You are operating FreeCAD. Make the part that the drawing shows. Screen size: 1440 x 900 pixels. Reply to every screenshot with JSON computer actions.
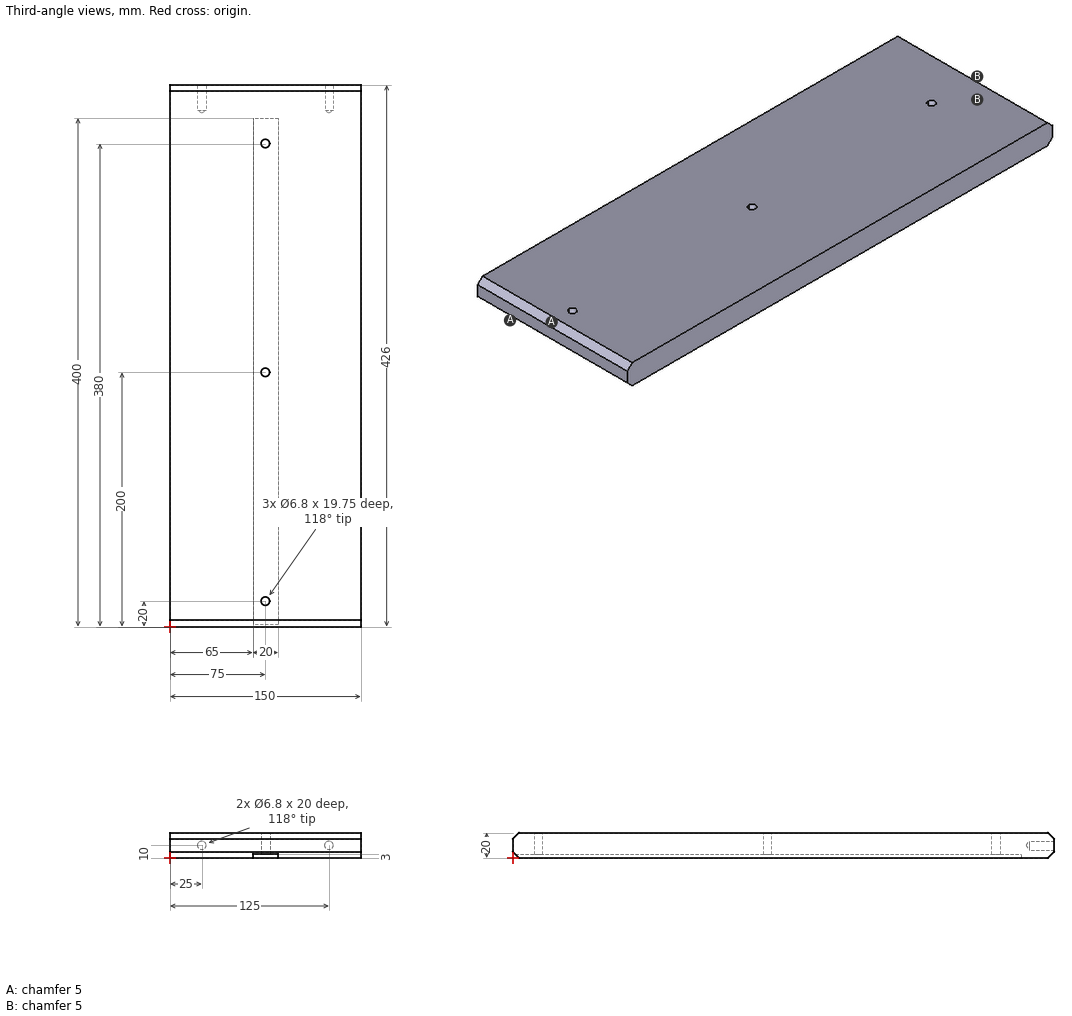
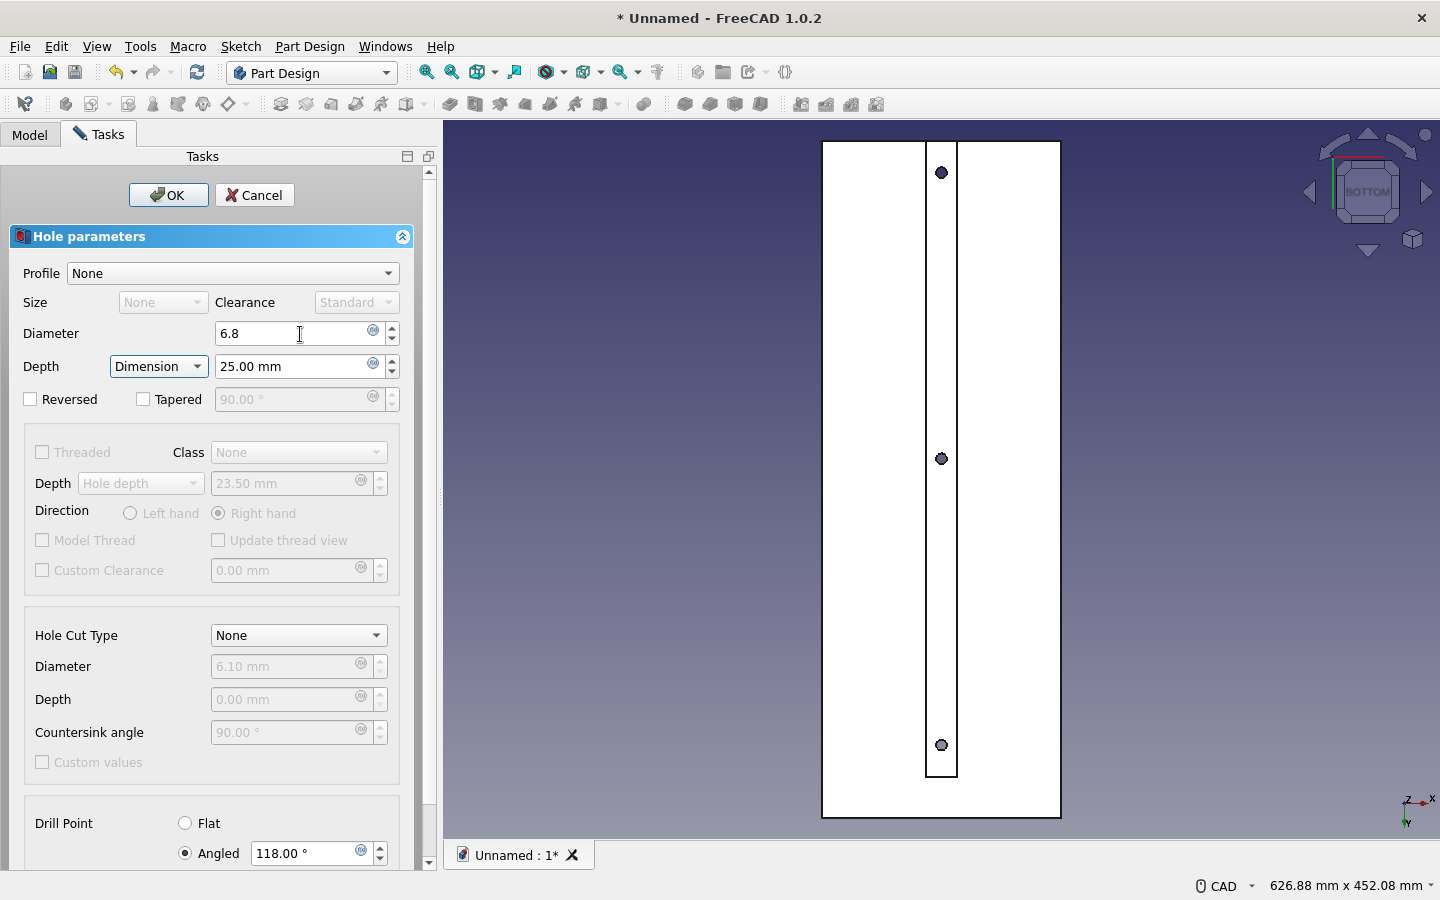
{"action": "triple_click", "coordinate": [300, 366]}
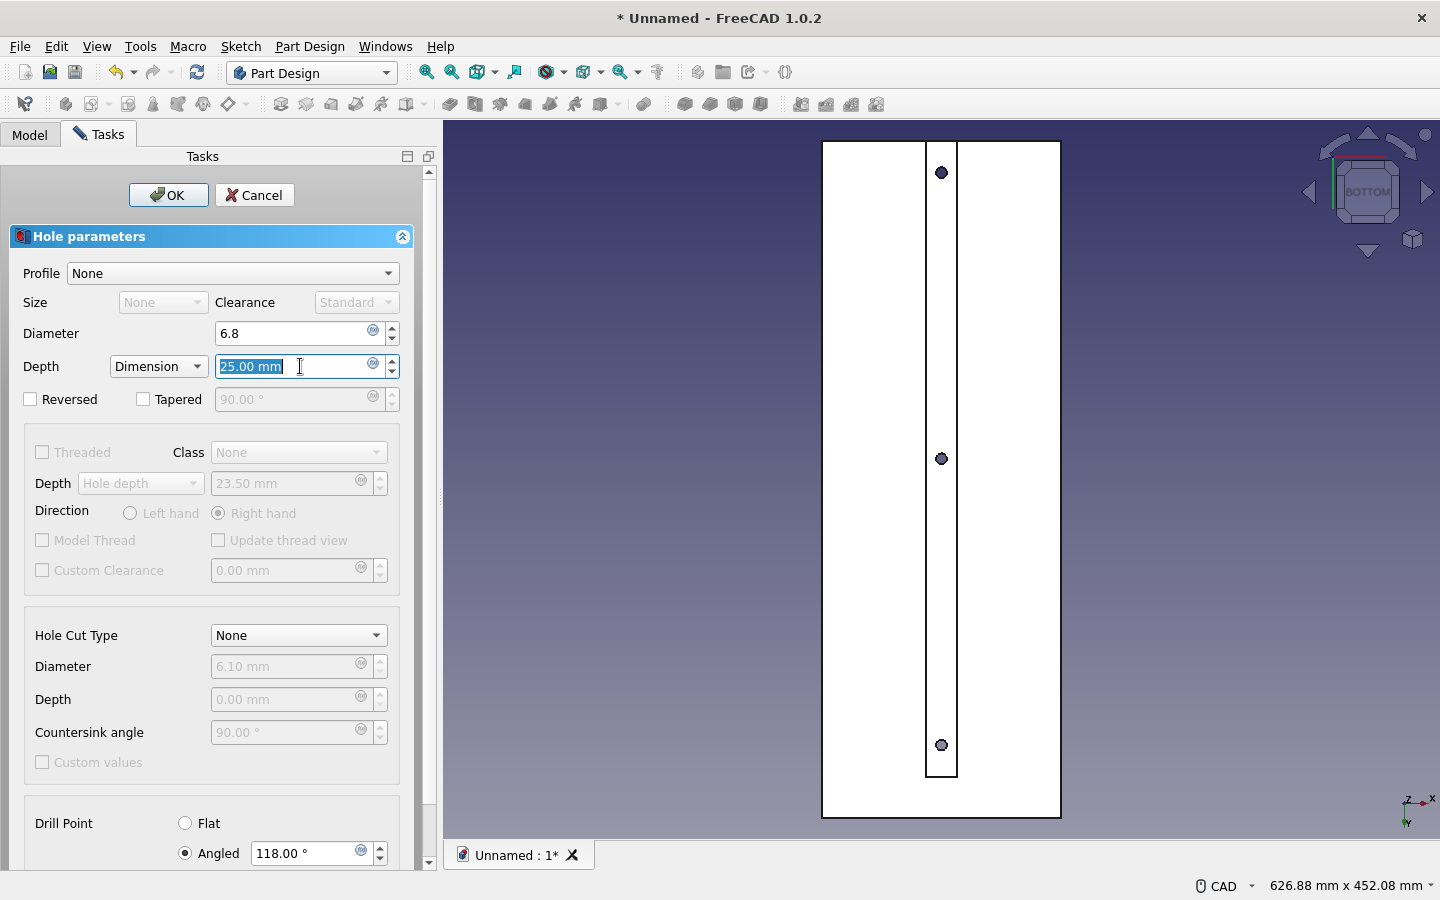
{"action": "type", "text": "19.75"}
{"action": "key", "text": "Tab"}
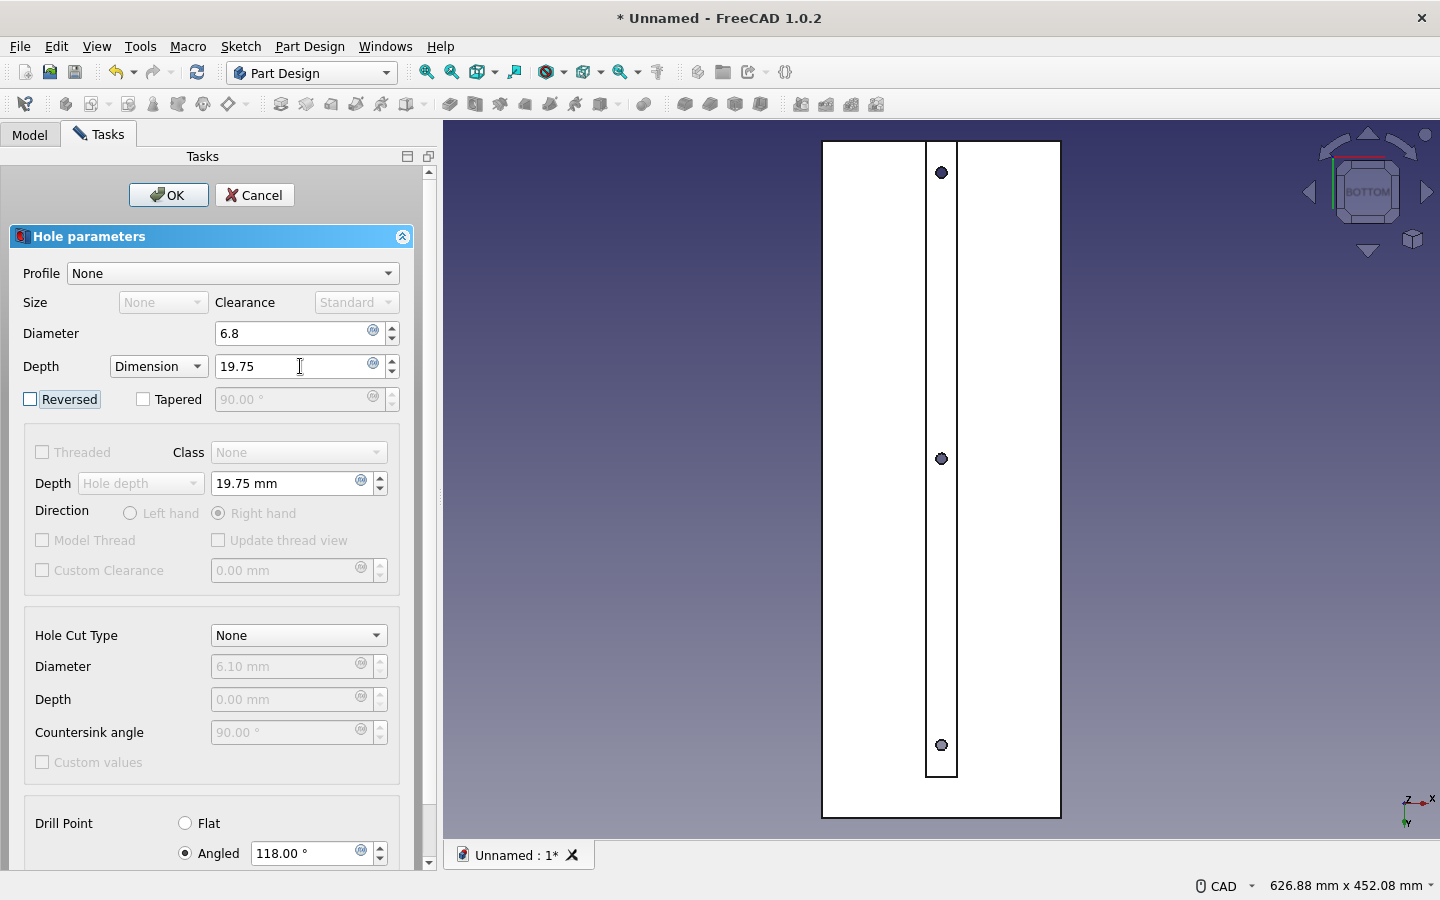
{"action": "left_click", "coordinate": [169, 195]}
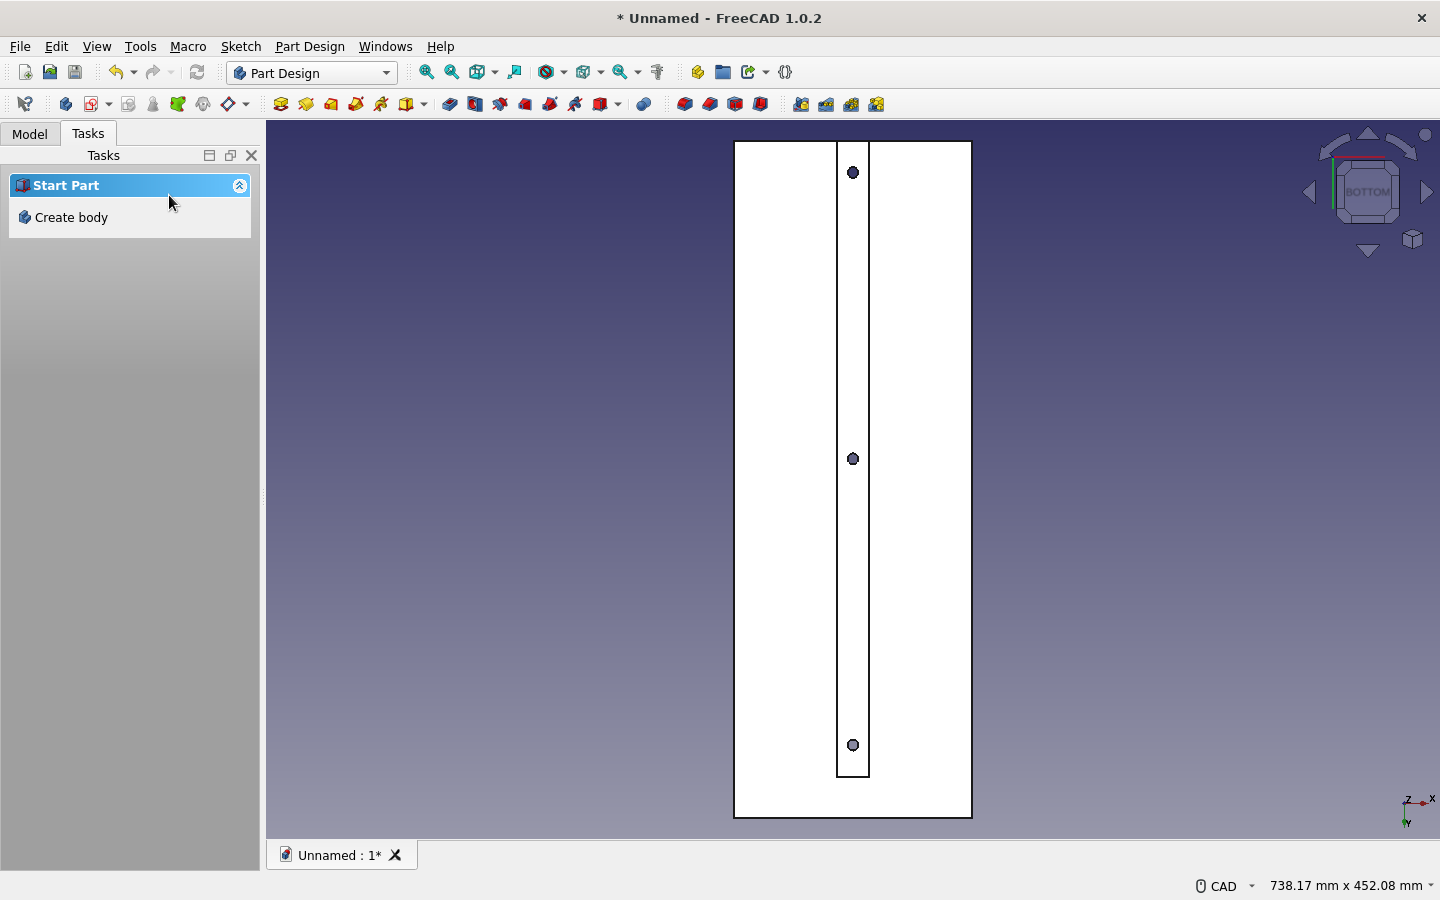
{"action": "key", "text": "4"}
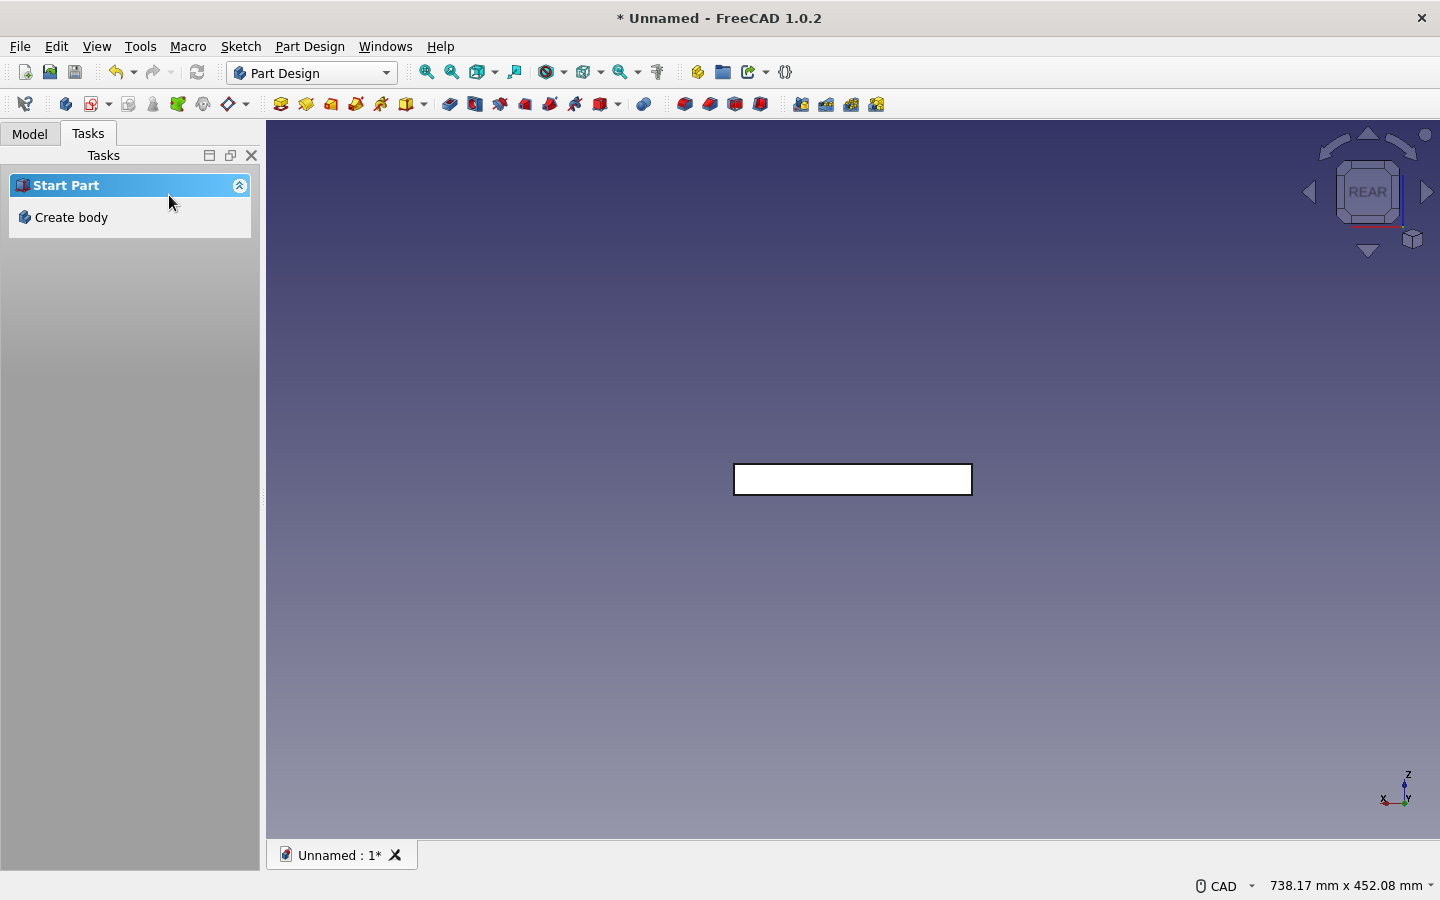
{"action": "key", "text": "v f"}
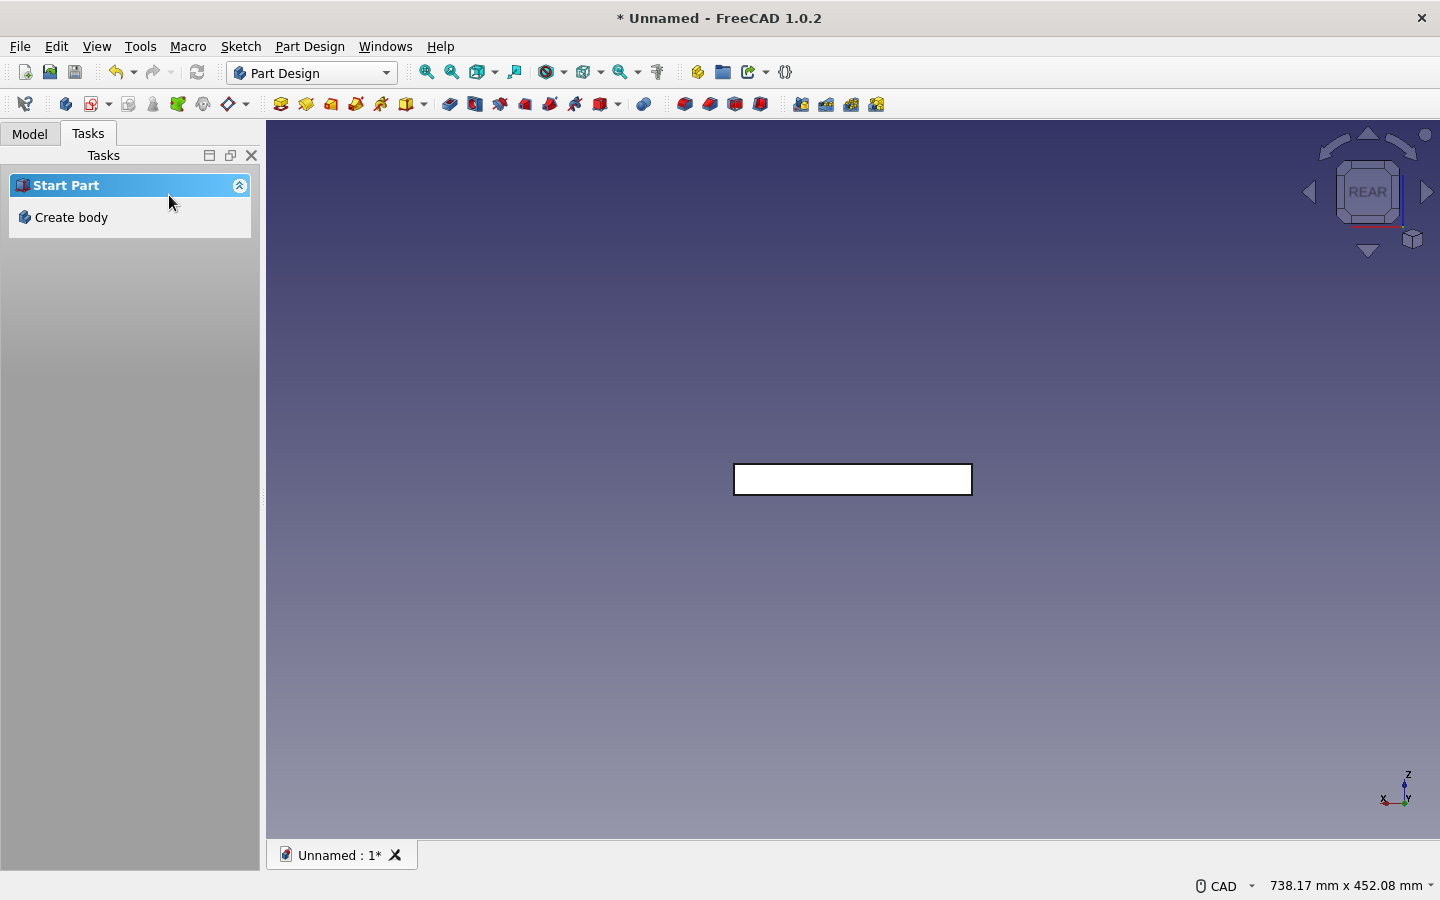
{"action": "left_click", "coordinate": [751, 479]}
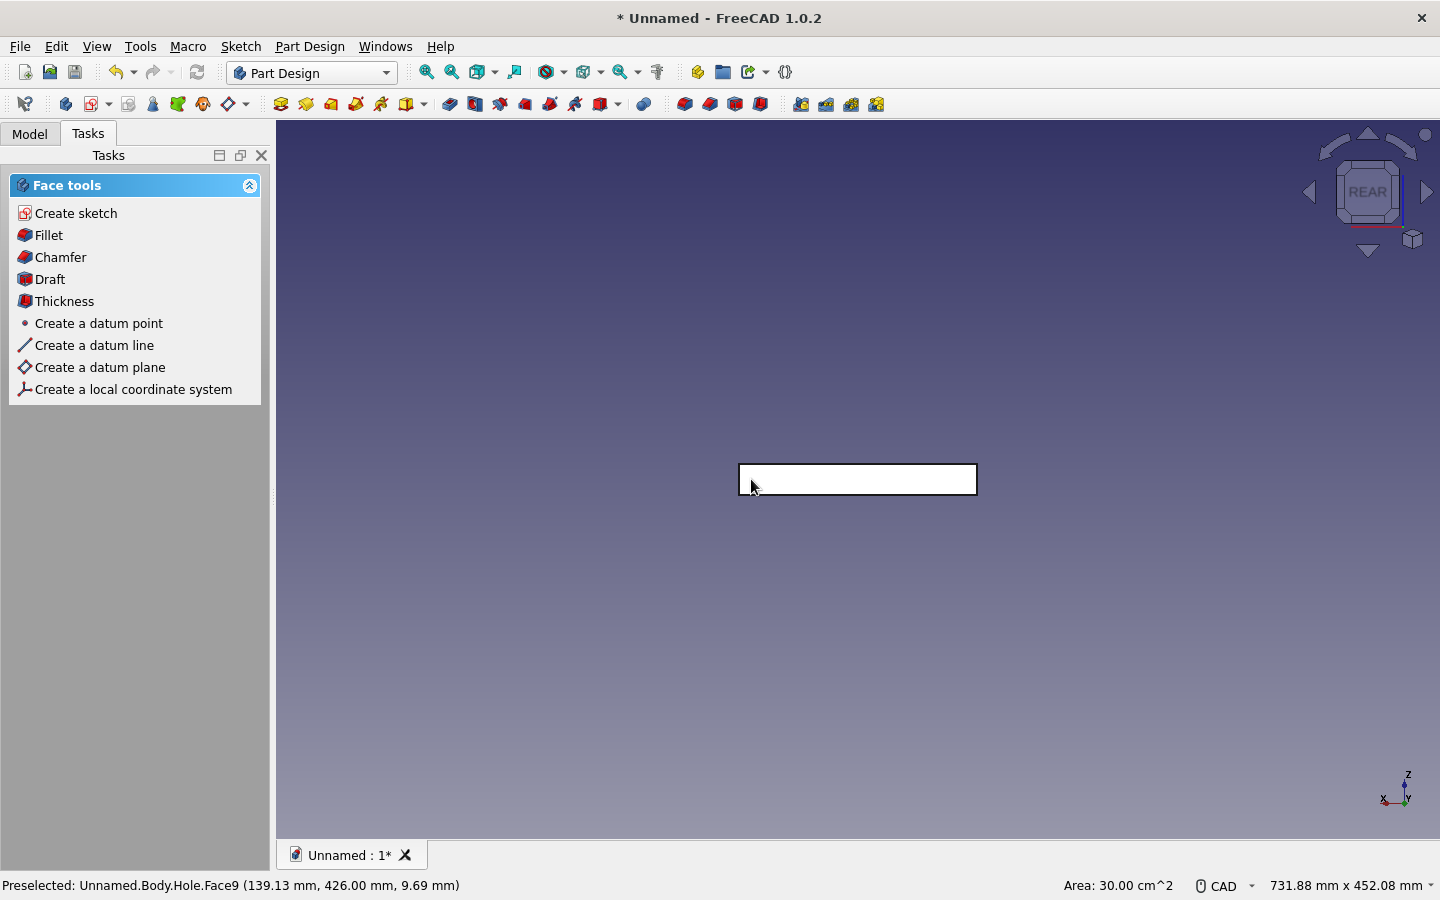
{"action": "left_click", "coordinate": [90, 104]}